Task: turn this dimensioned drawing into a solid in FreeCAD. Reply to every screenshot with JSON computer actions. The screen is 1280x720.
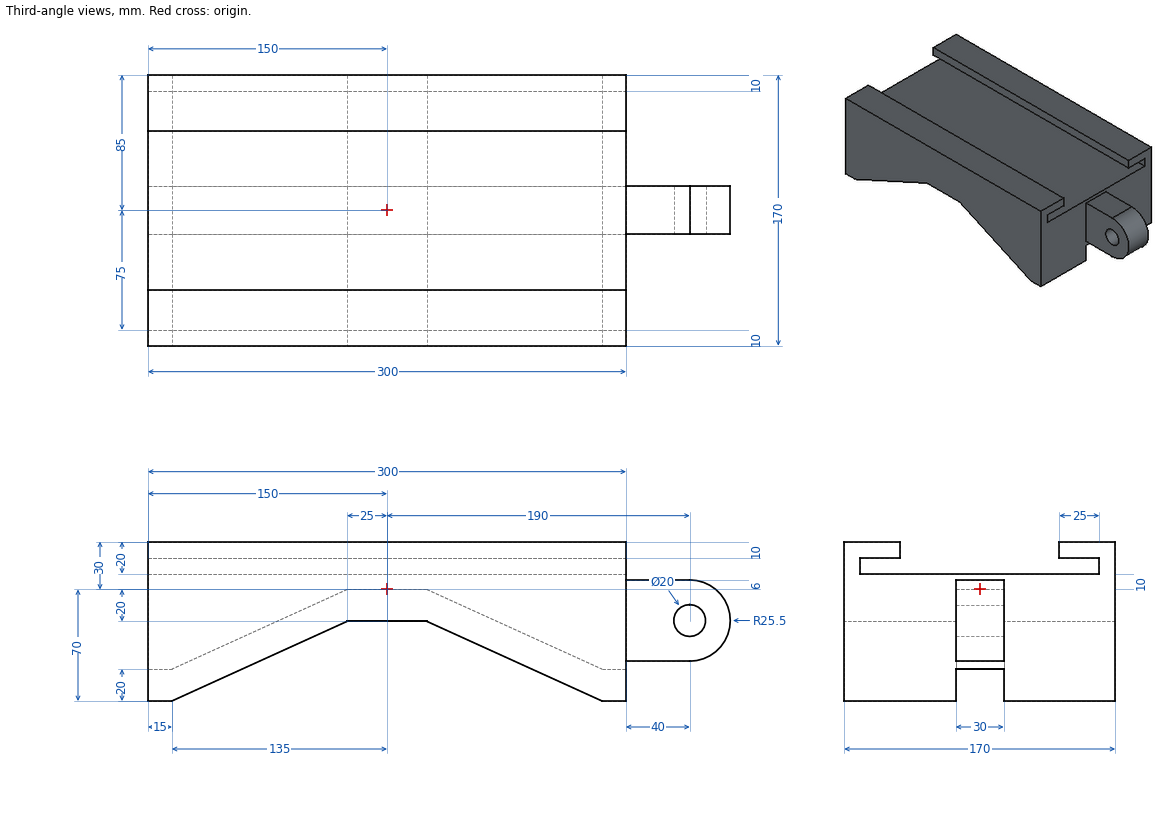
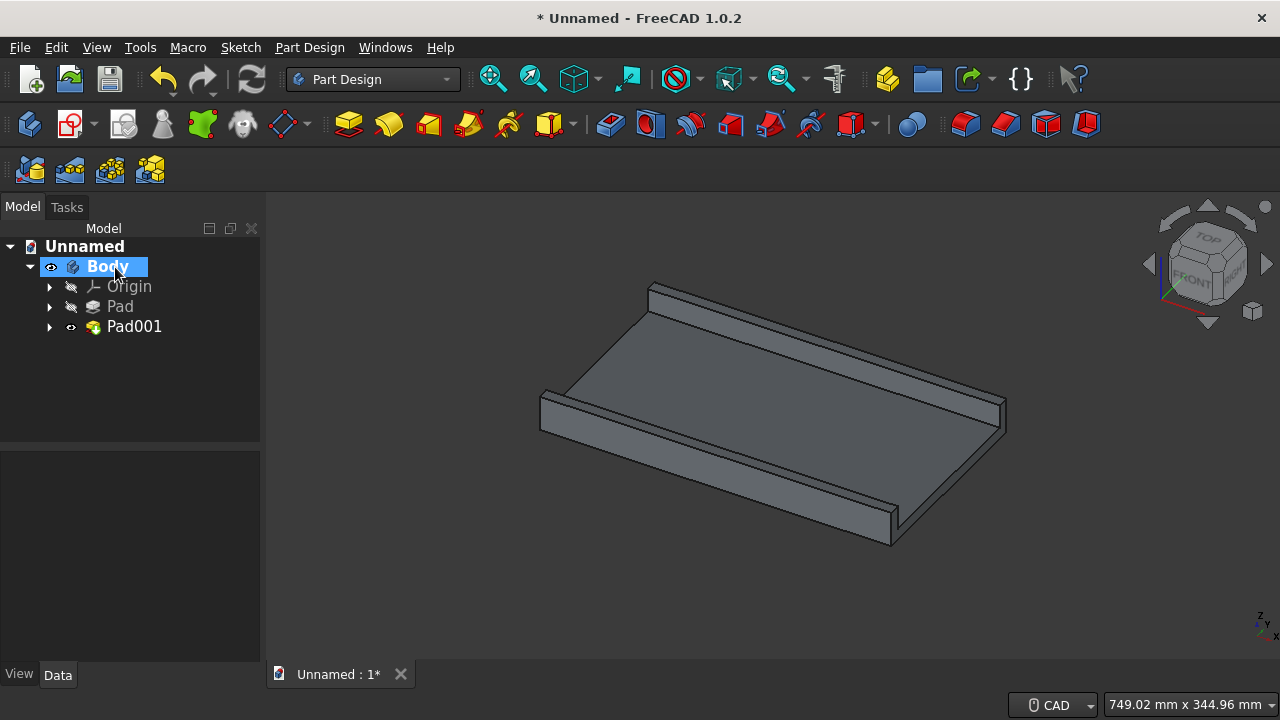
{"action": "left_click", "coordinate": [50, 287]}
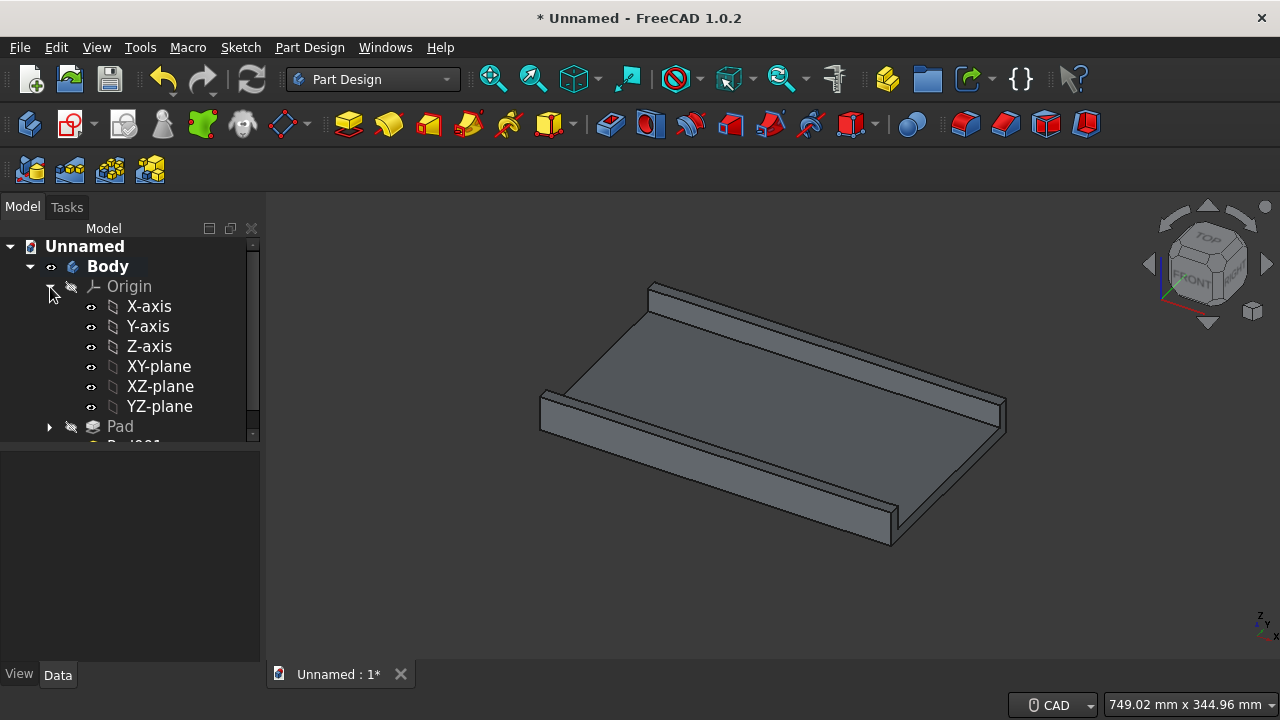
{"action": "left_click", "coordinate": [136, 387]}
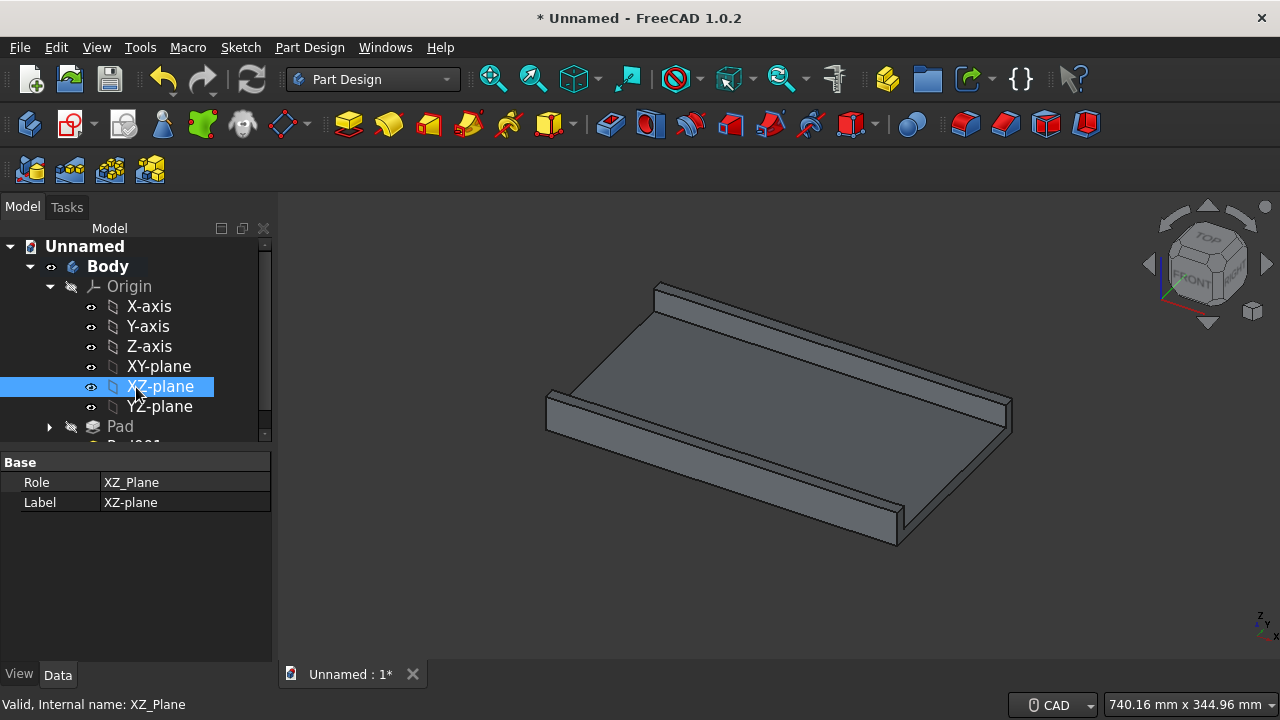
{"action": "left_click", "coordinate": [284, 124]}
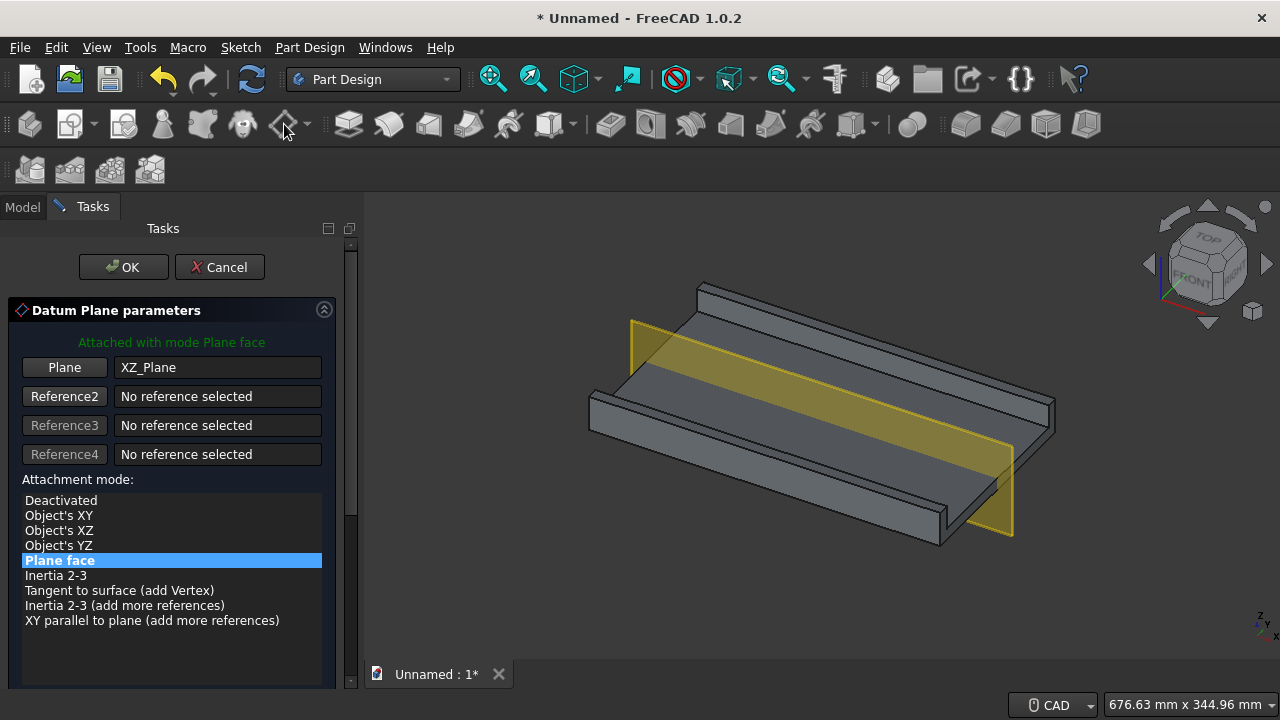
{"action": "scroll", "coordinate": [351, 463], "scroll_direction": "down", "scroll_amount": 3}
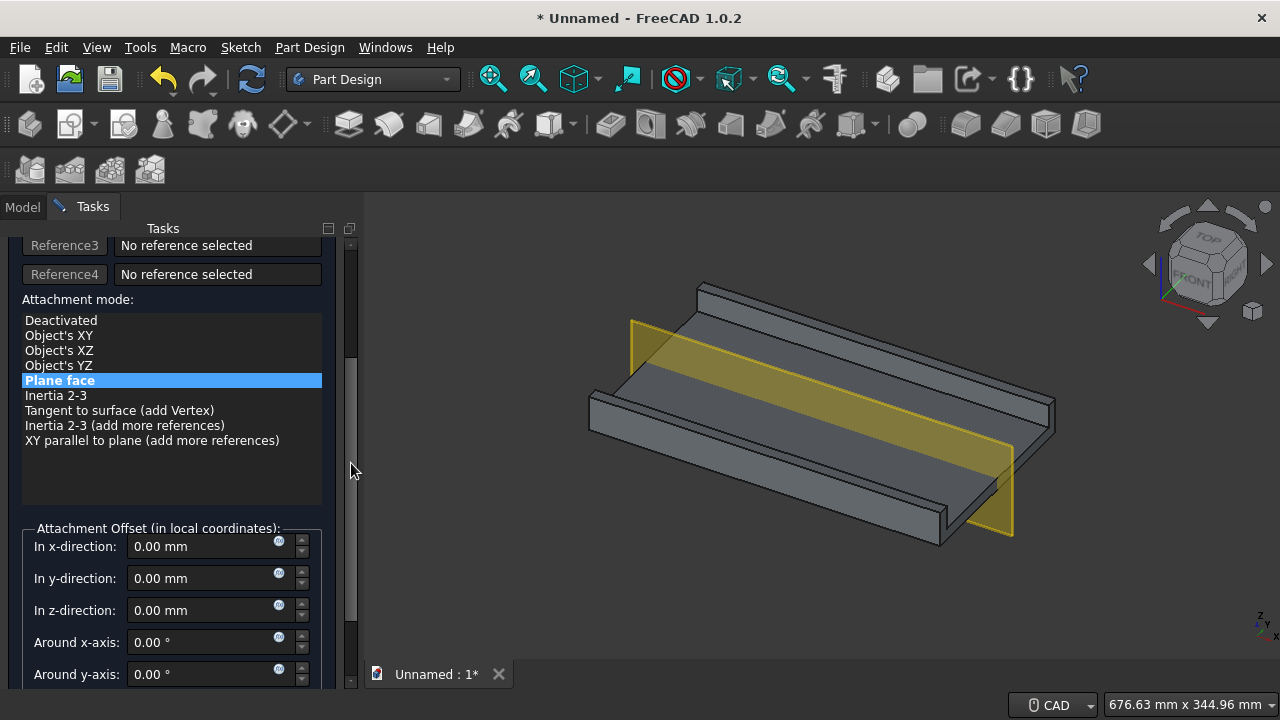
{"action": "triple_click", "coordinate": [210, 610]}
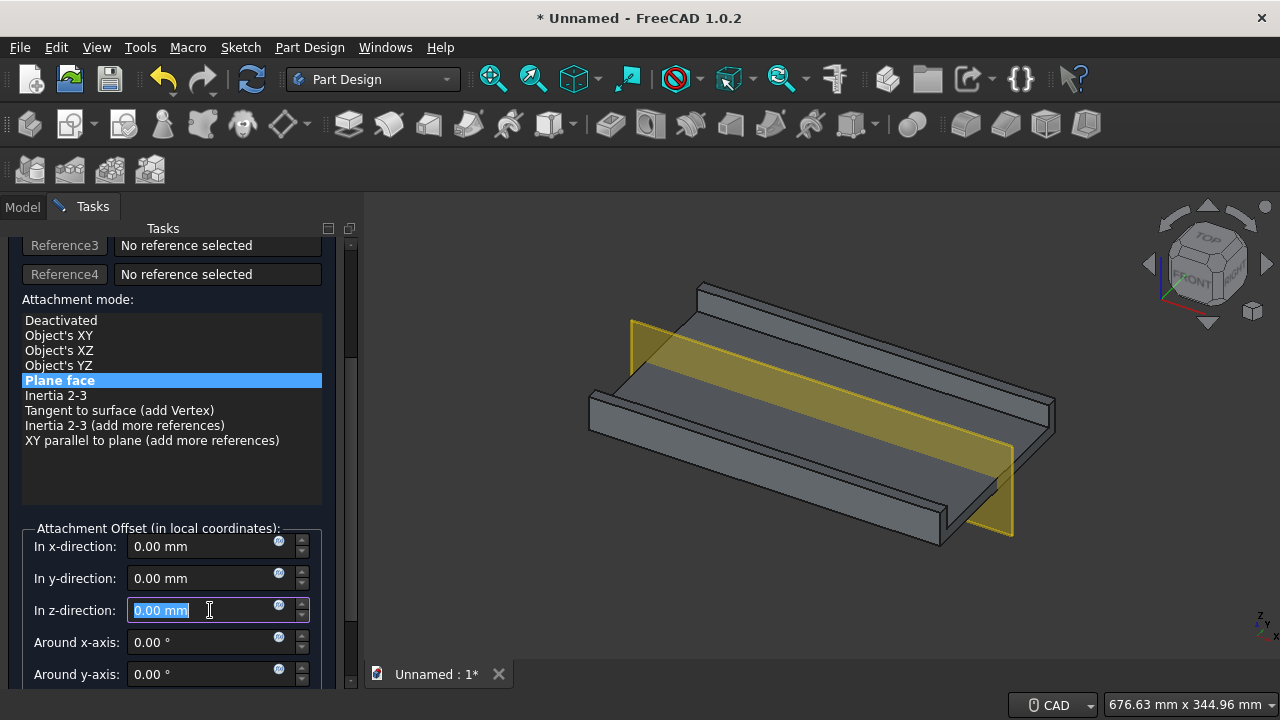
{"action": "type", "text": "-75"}
{"action": "key", "text": "Tab"}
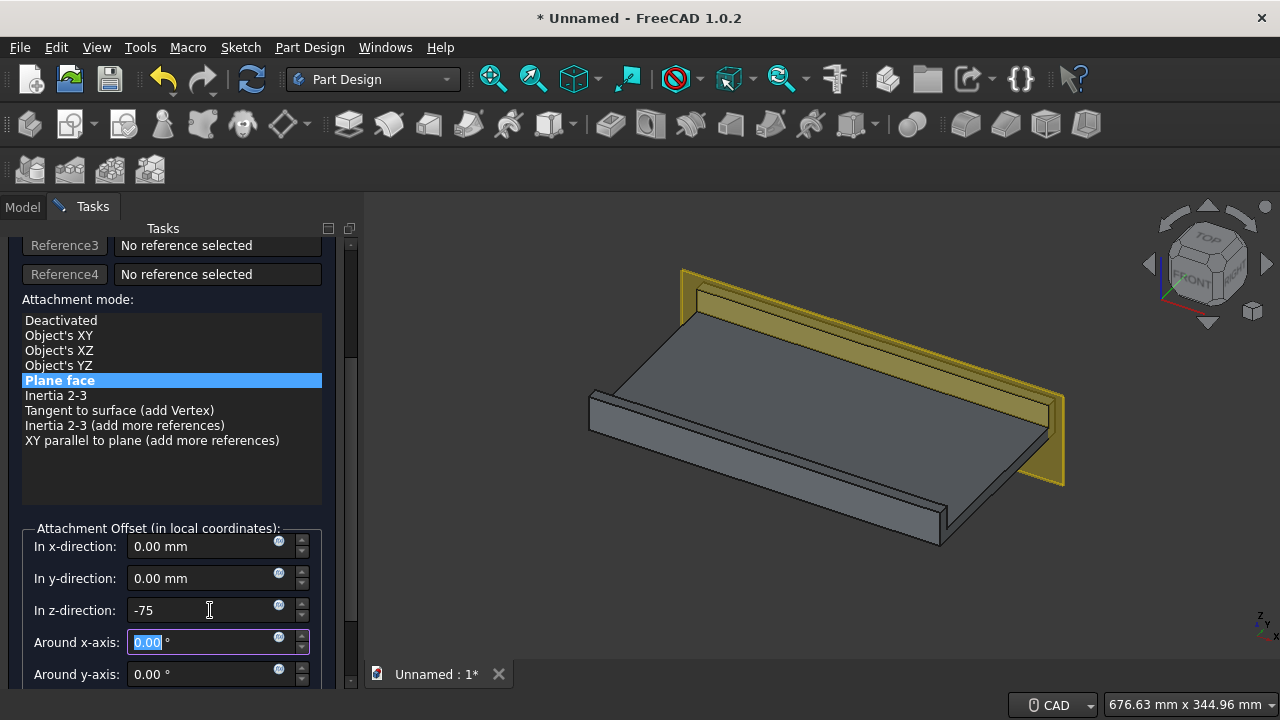
{"action": "scroll", "coordinate": [351, 463], "scroll_direction": "up", "scroll_amount": 4}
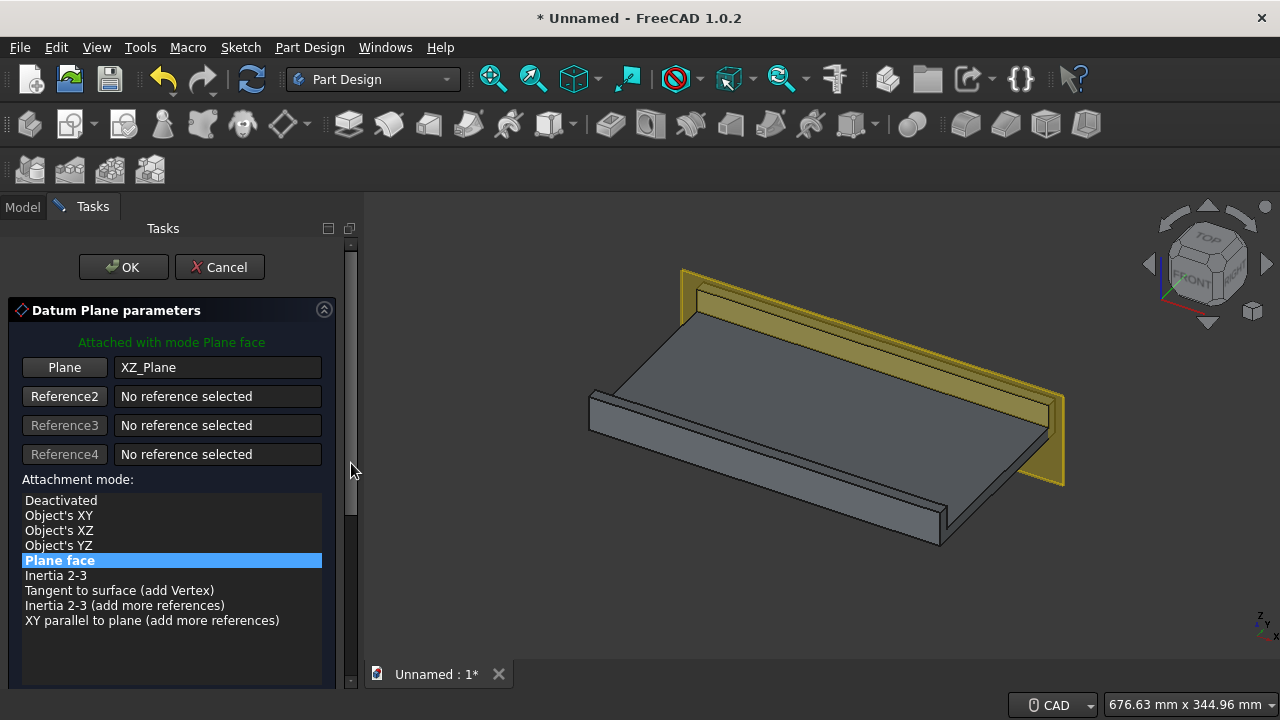
{"action": "left_click", "coordinate": [124, 267]}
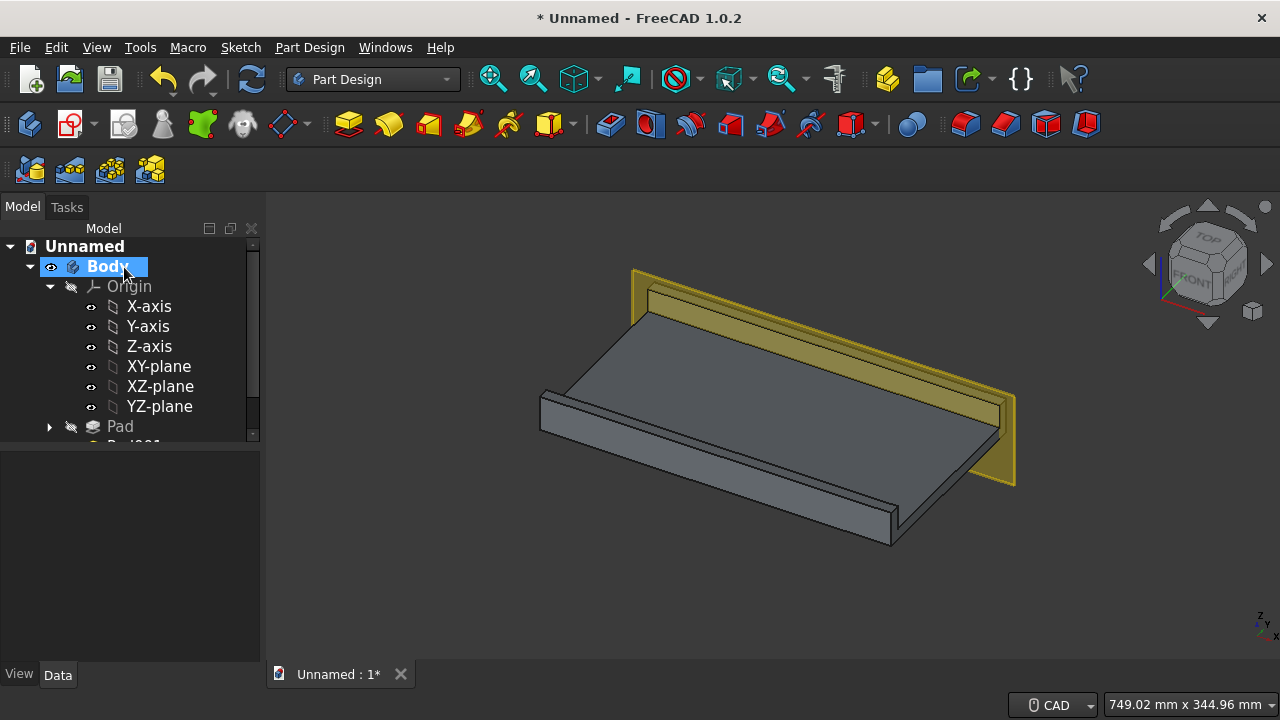
{"action": "scroll", "coordinate": [100, 342], "scroll_direction": "down", "scroll_amount": 3}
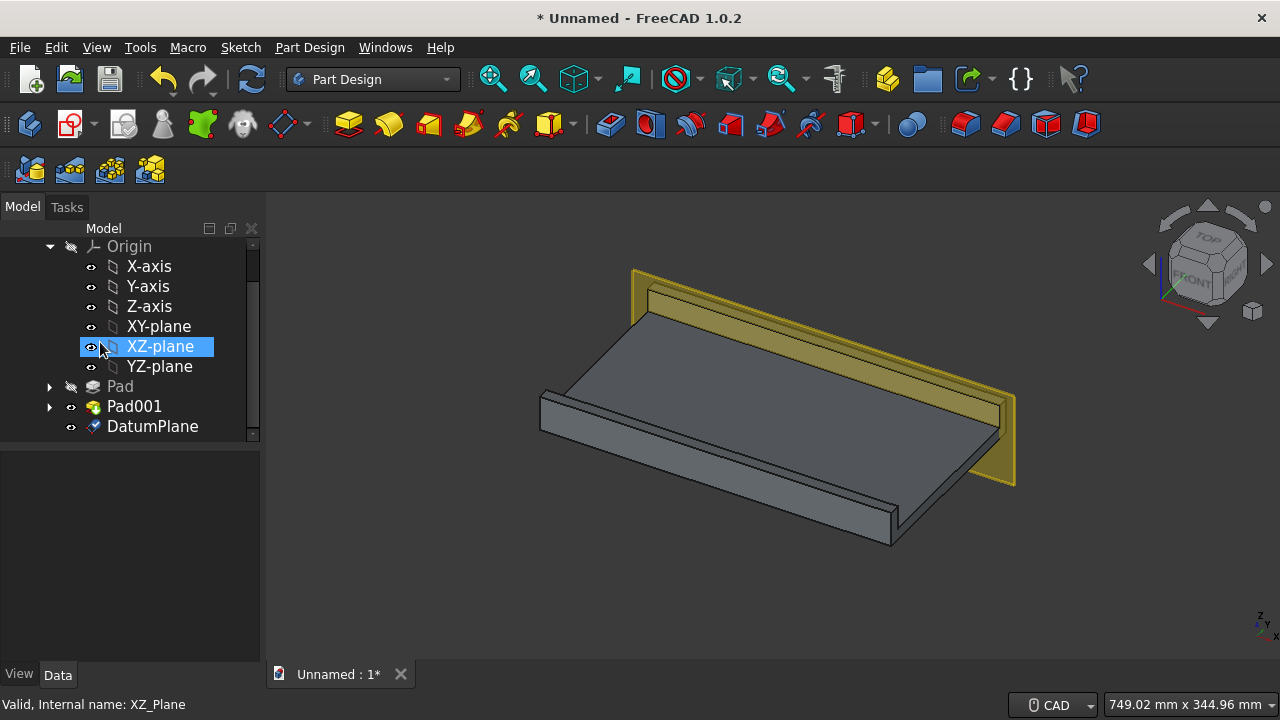
{"action": "left_click", "coordinate": [116, 427]}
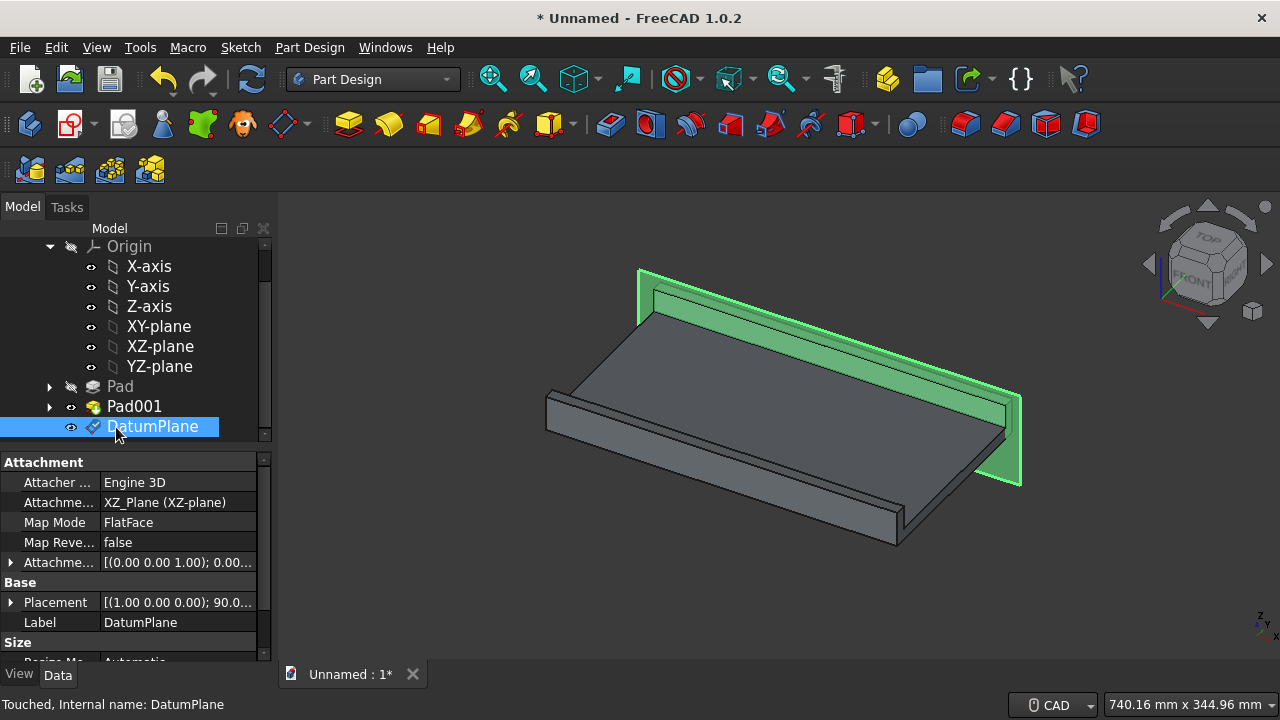
{"action": "left_click", "coordinate": [70, 124]}